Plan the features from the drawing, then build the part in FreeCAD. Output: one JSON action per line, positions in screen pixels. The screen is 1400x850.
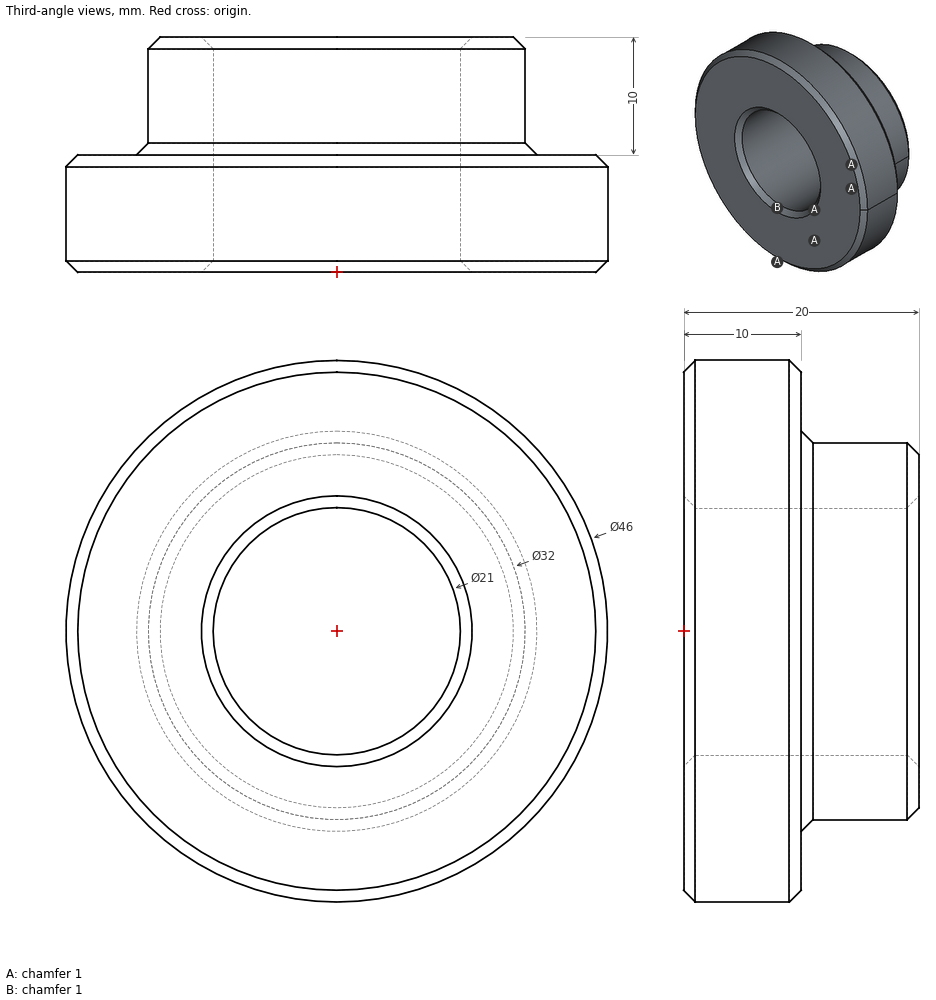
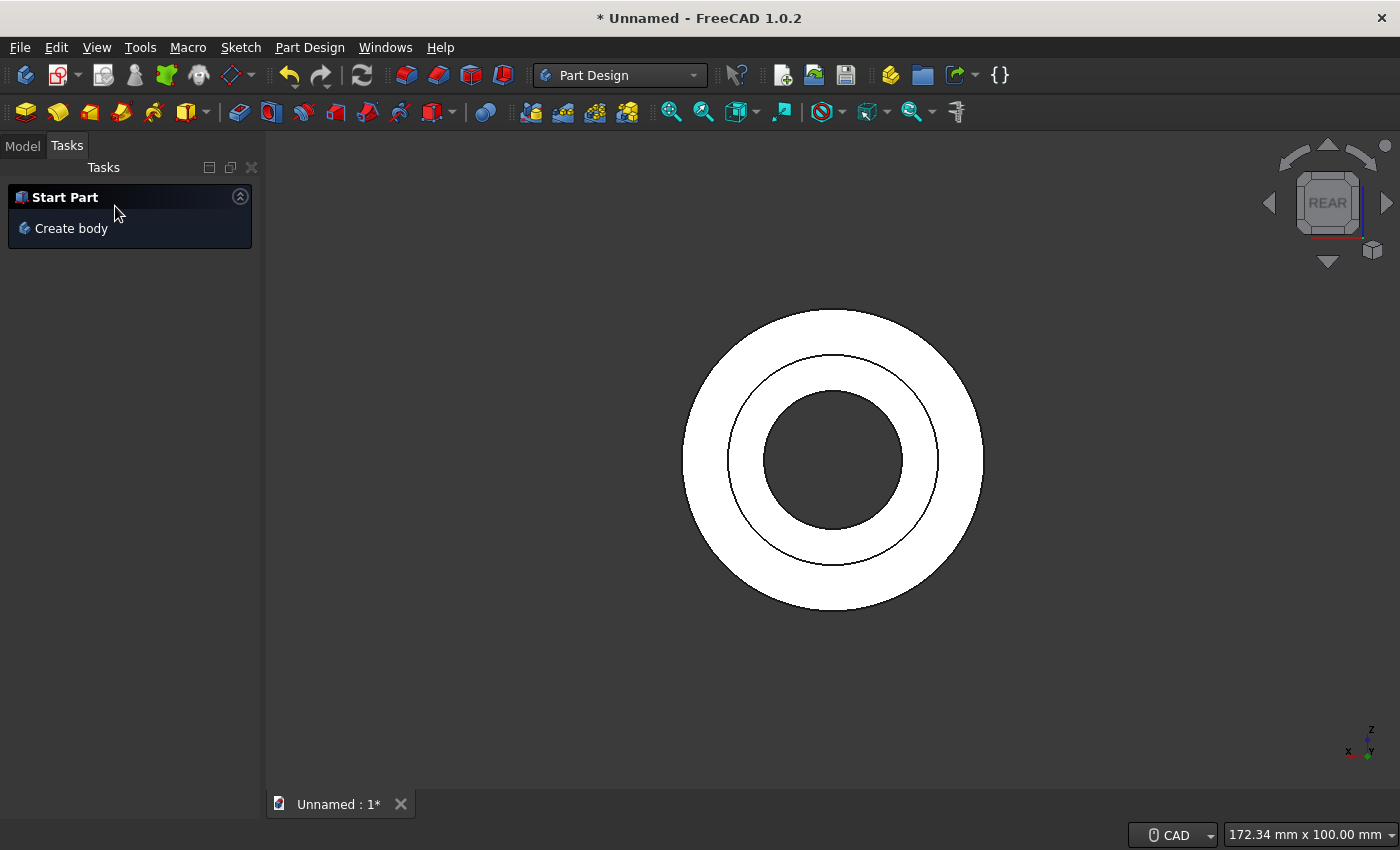
{"action": "left_click", "coordinate": [889, 418]}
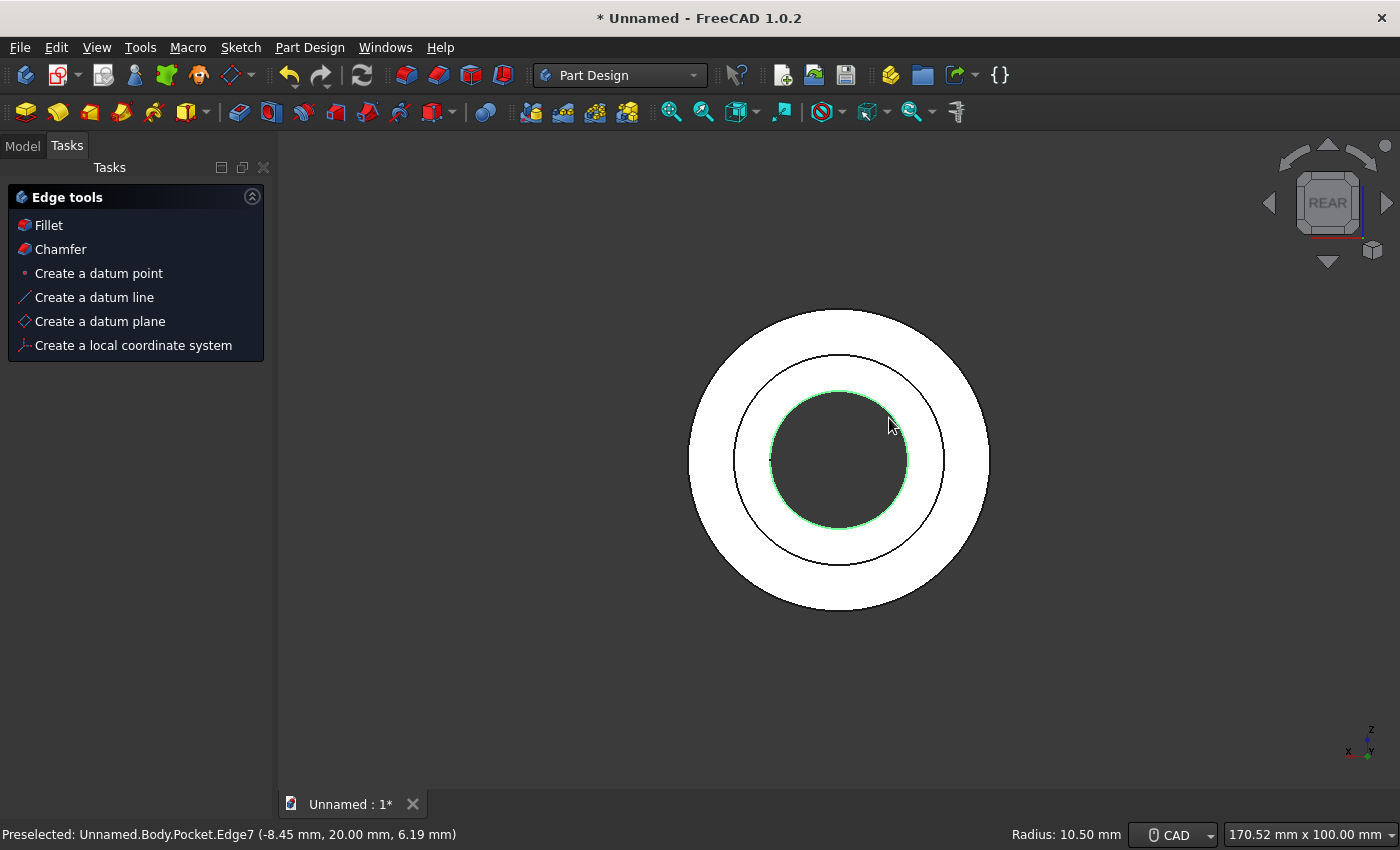
{"action": "left_click", "coordinate": [990, 459], "text": "ctrl"}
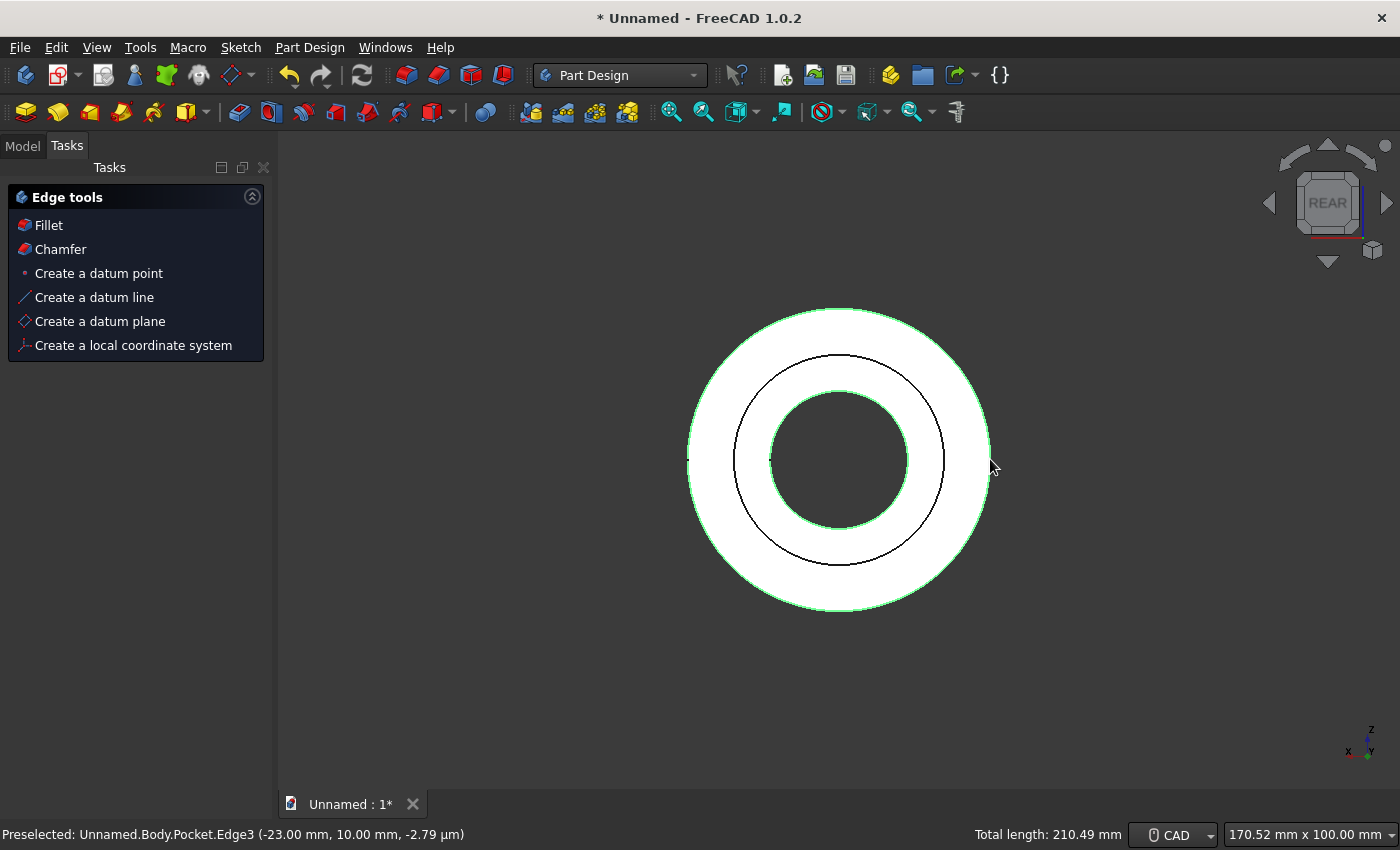
{"action": "left_click", "coordinate": [944, 459], "text": "ctrl"}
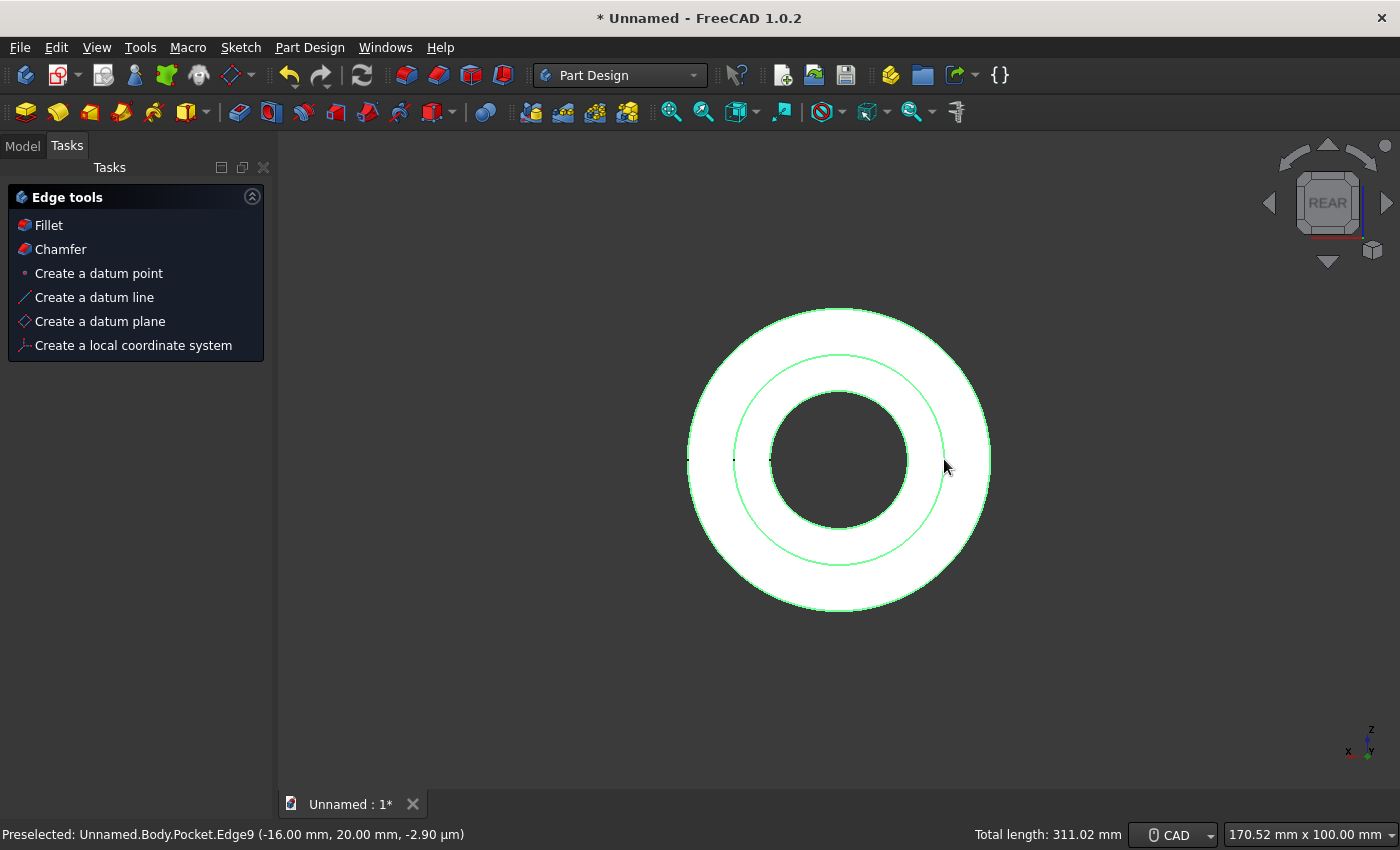
{"action": "key", "text": "0"}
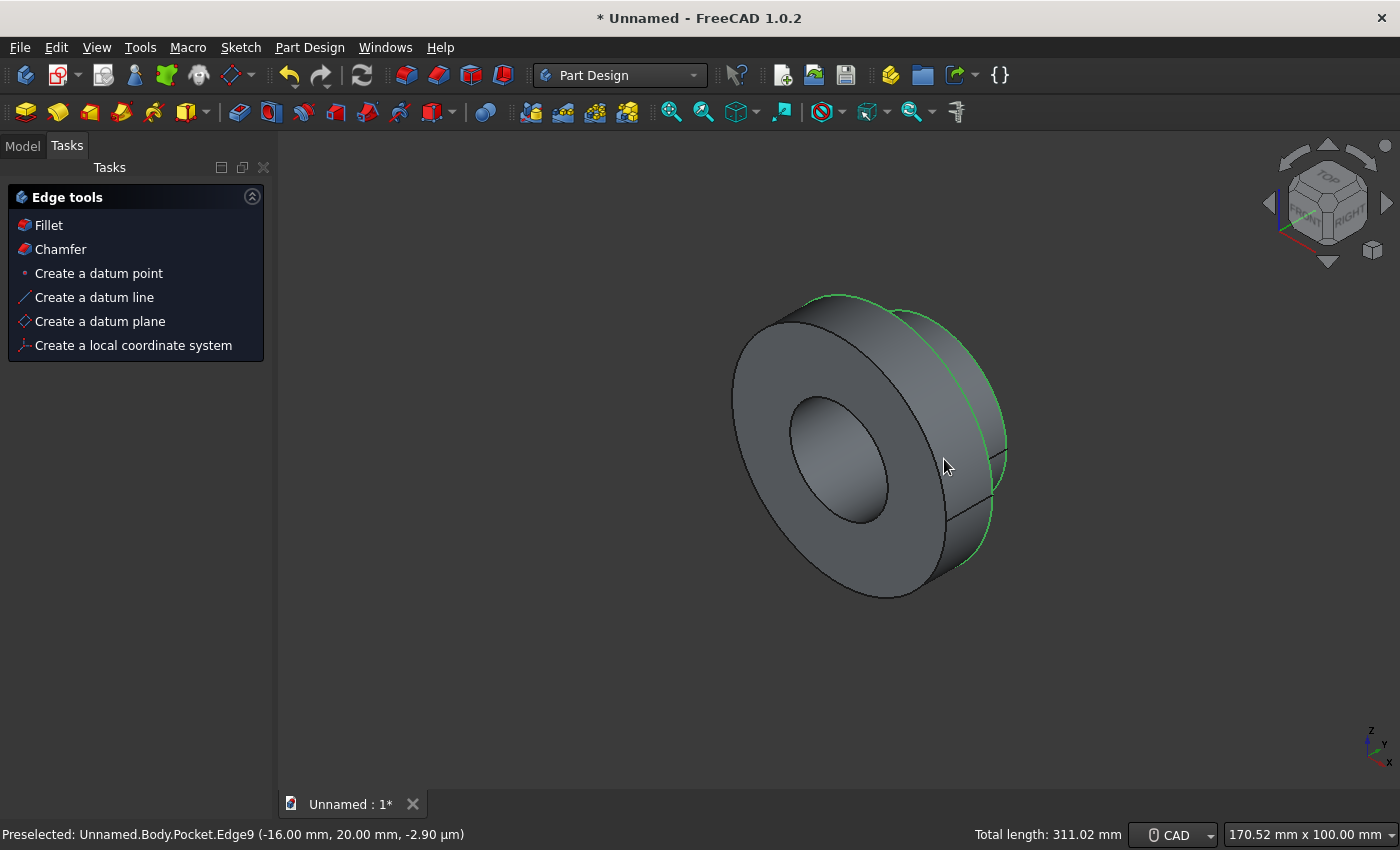
{"action": "left_click", "coordinate": [752, 336], "text": "ctrl"}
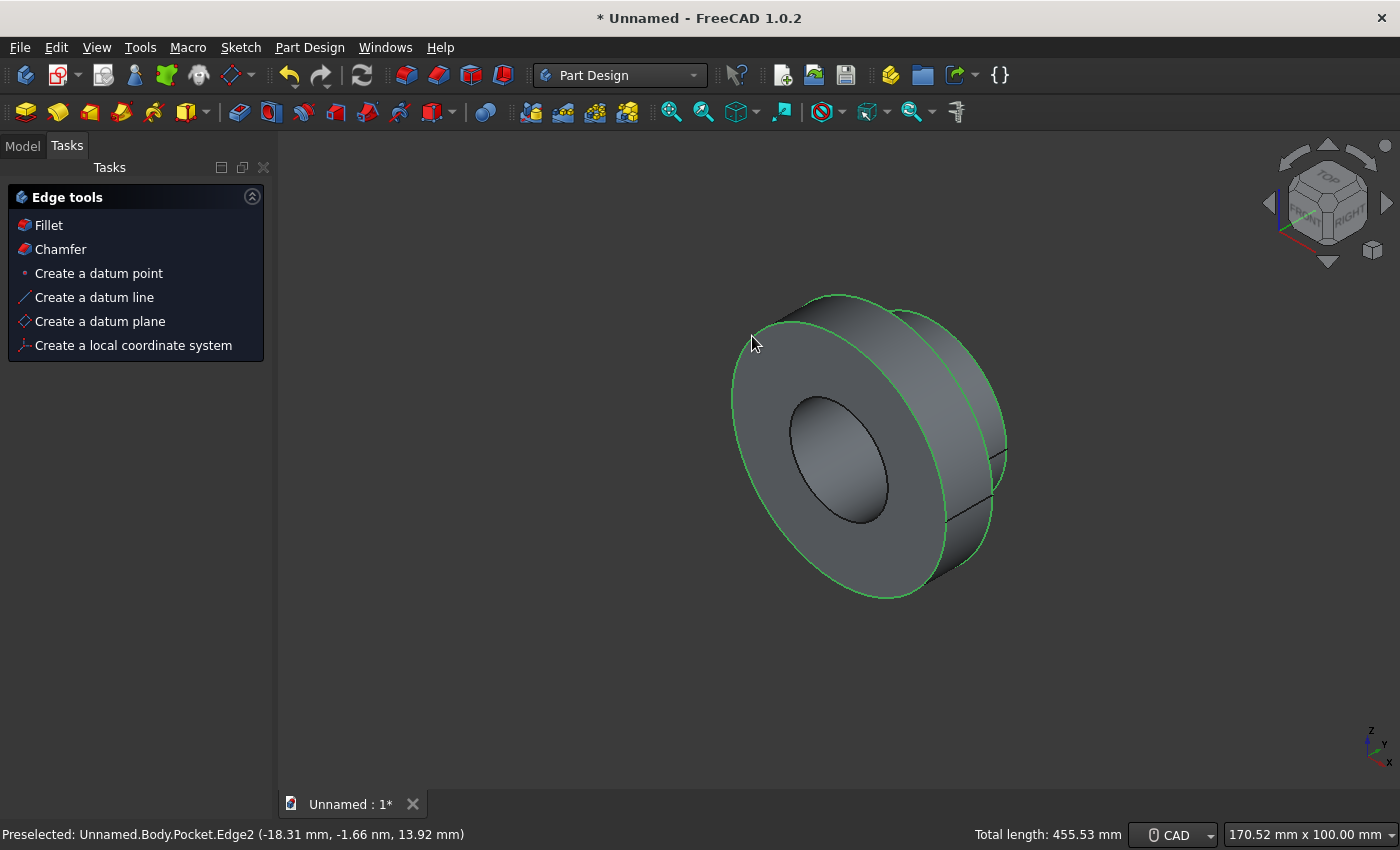
{"action": "key", "text": "2"}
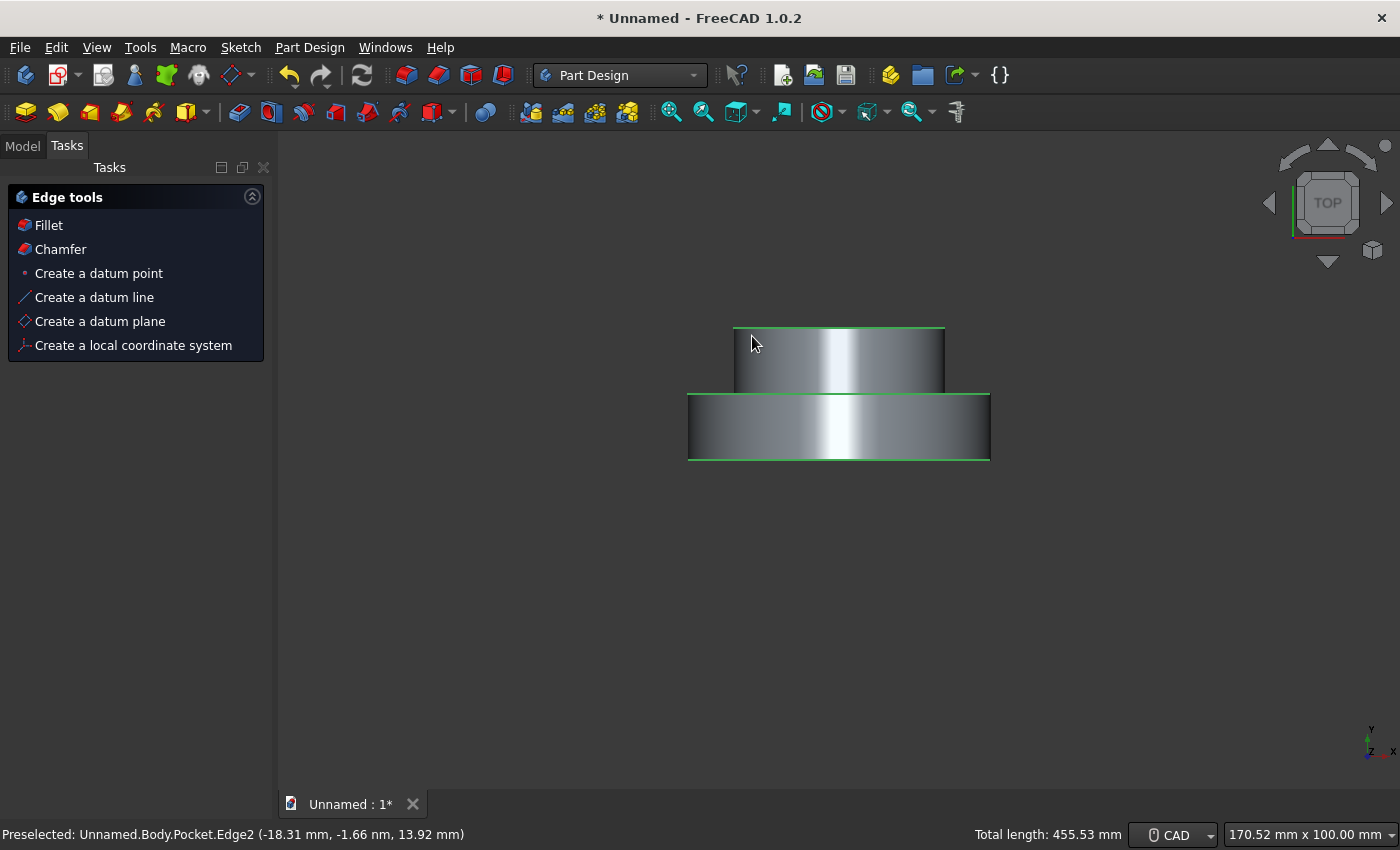
{"action": "key", "text": "v f"}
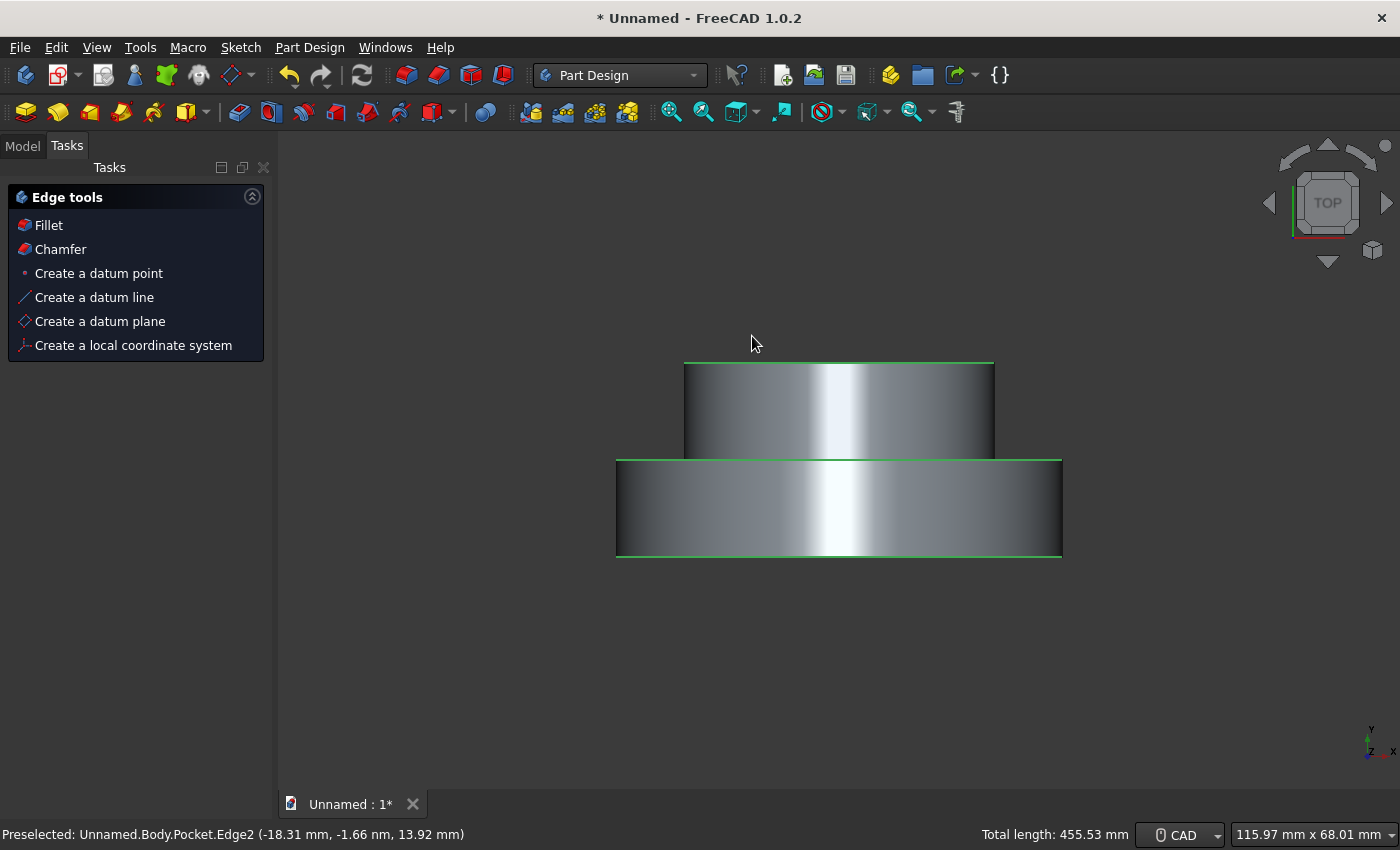
{"action": "key", "text": "1"}